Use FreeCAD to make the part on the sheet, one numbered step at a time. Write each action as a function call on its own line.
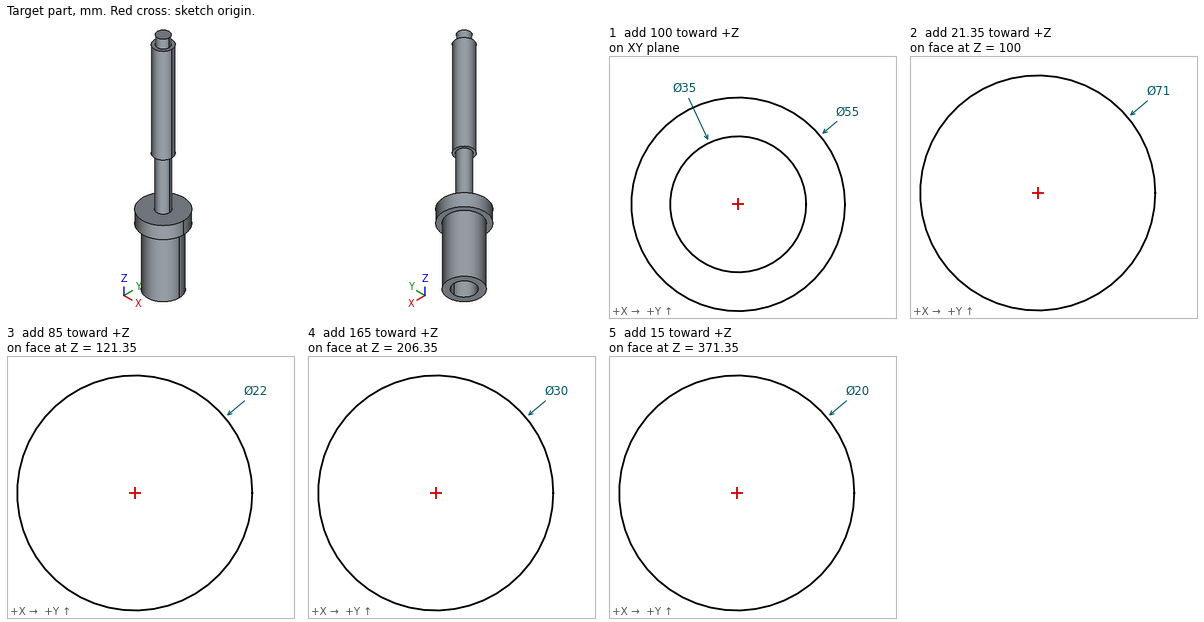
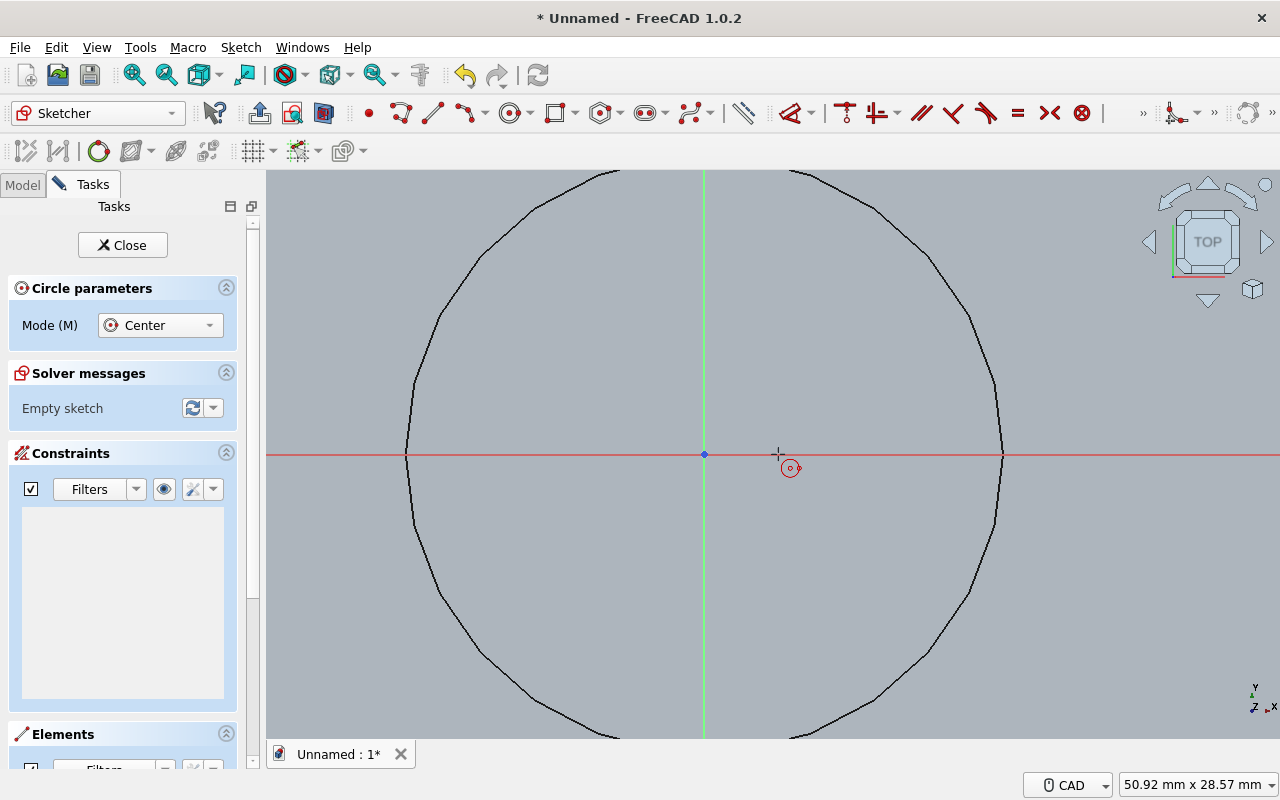
click(704, 454)
click(845, 314)
key(Escape)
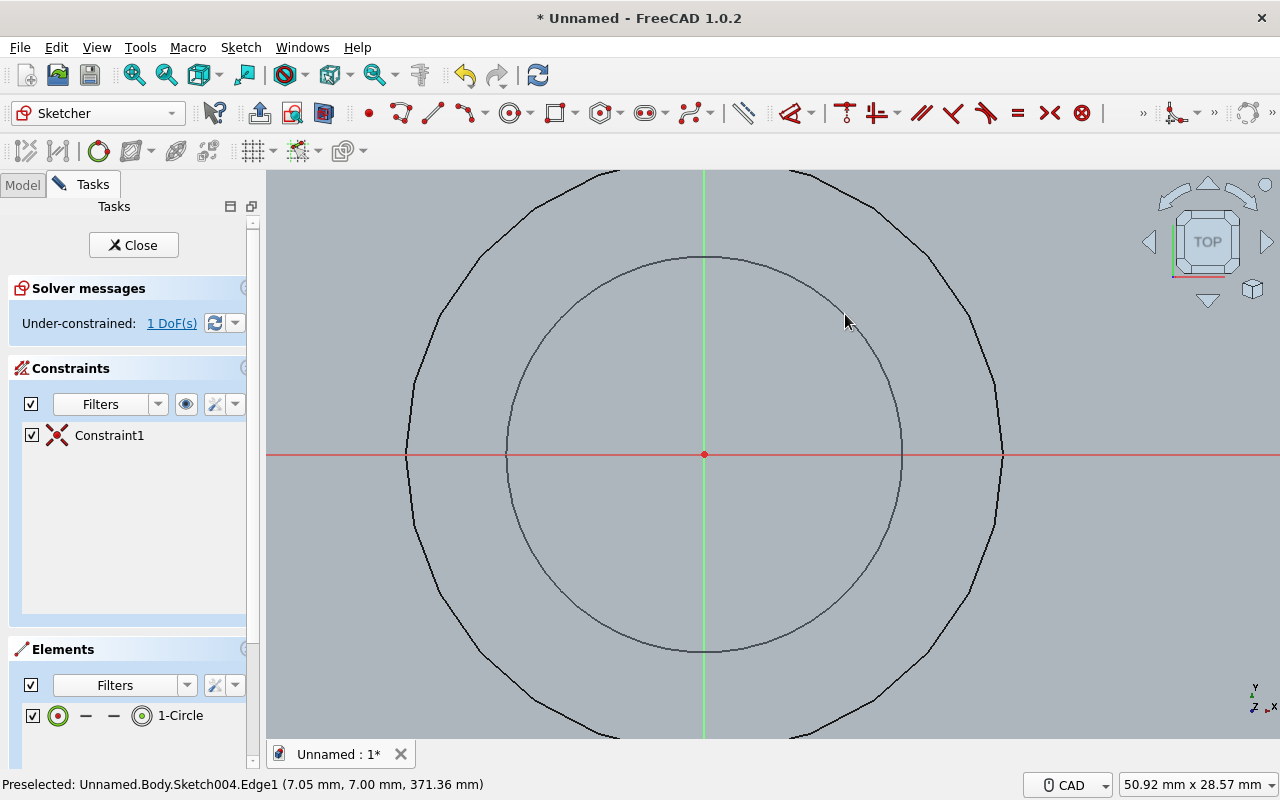
click(844, 314)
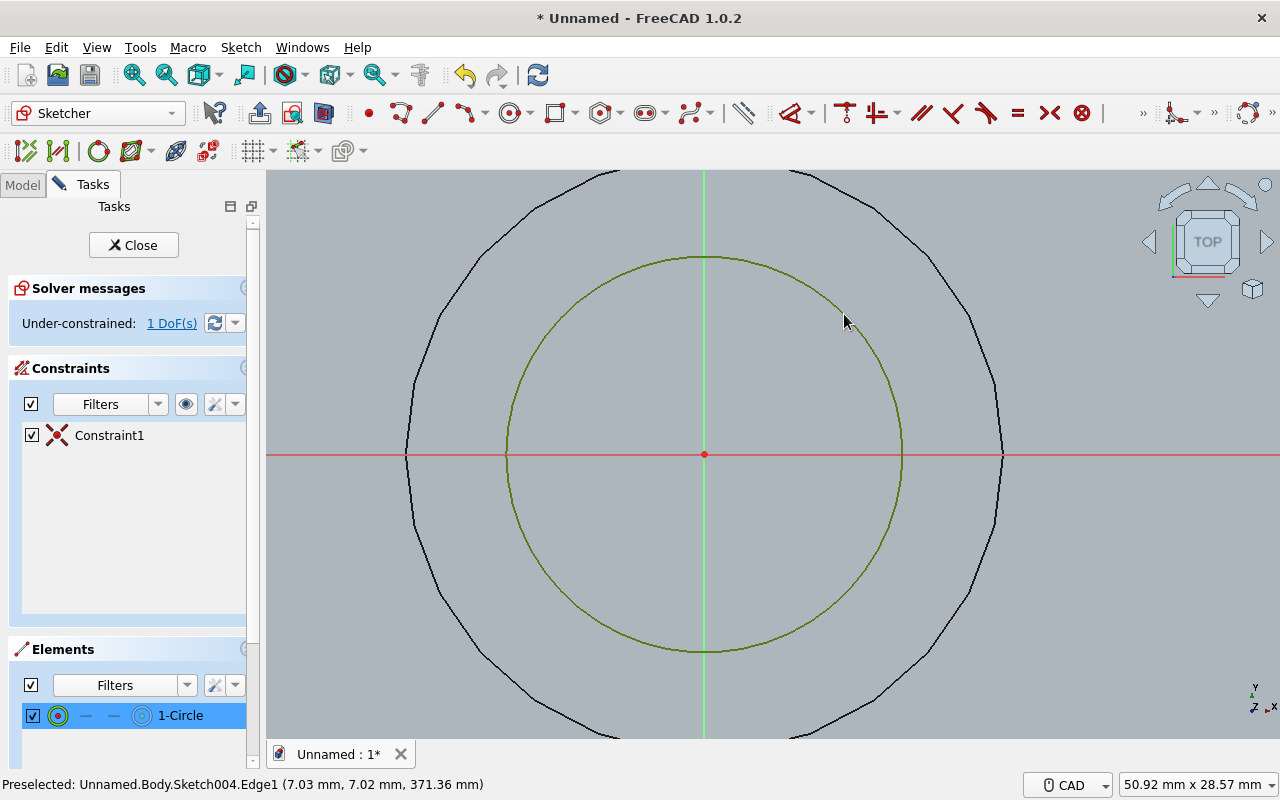
key(k)
key(o)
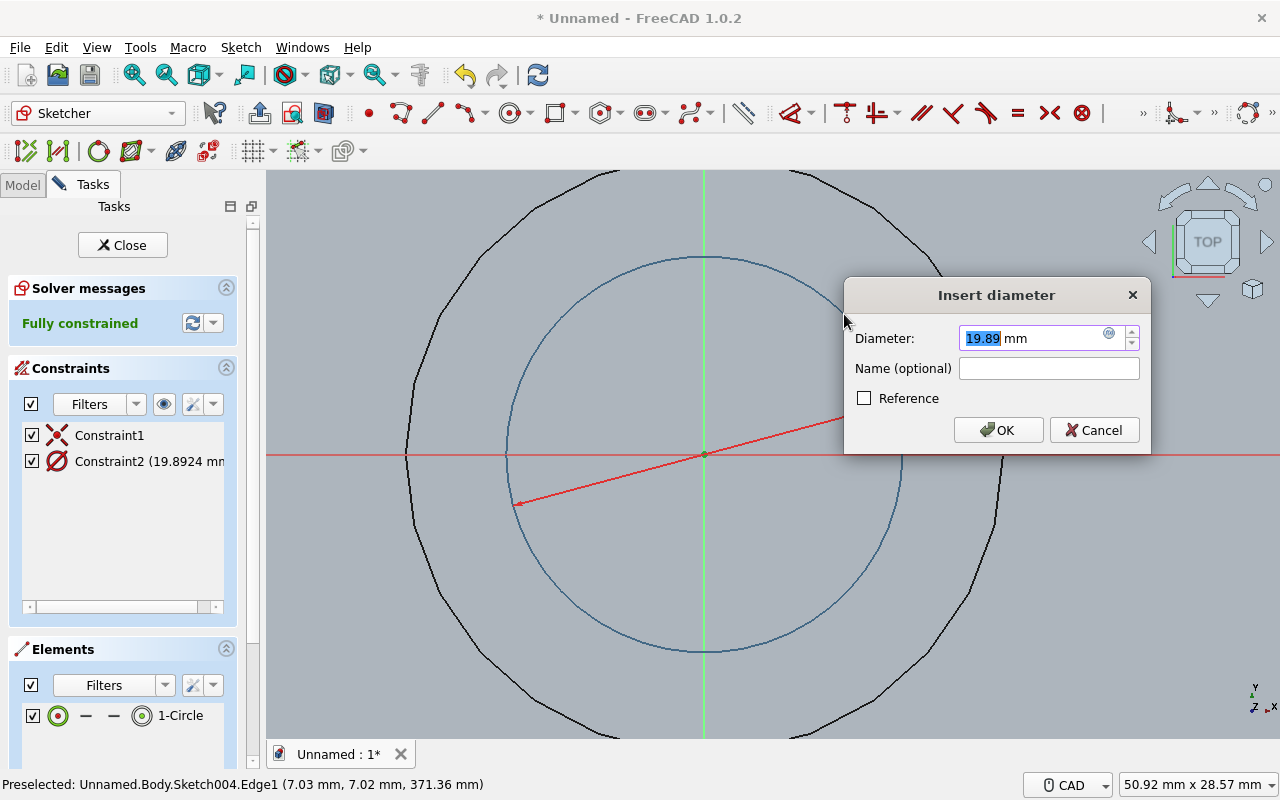
text(20)
key(Return)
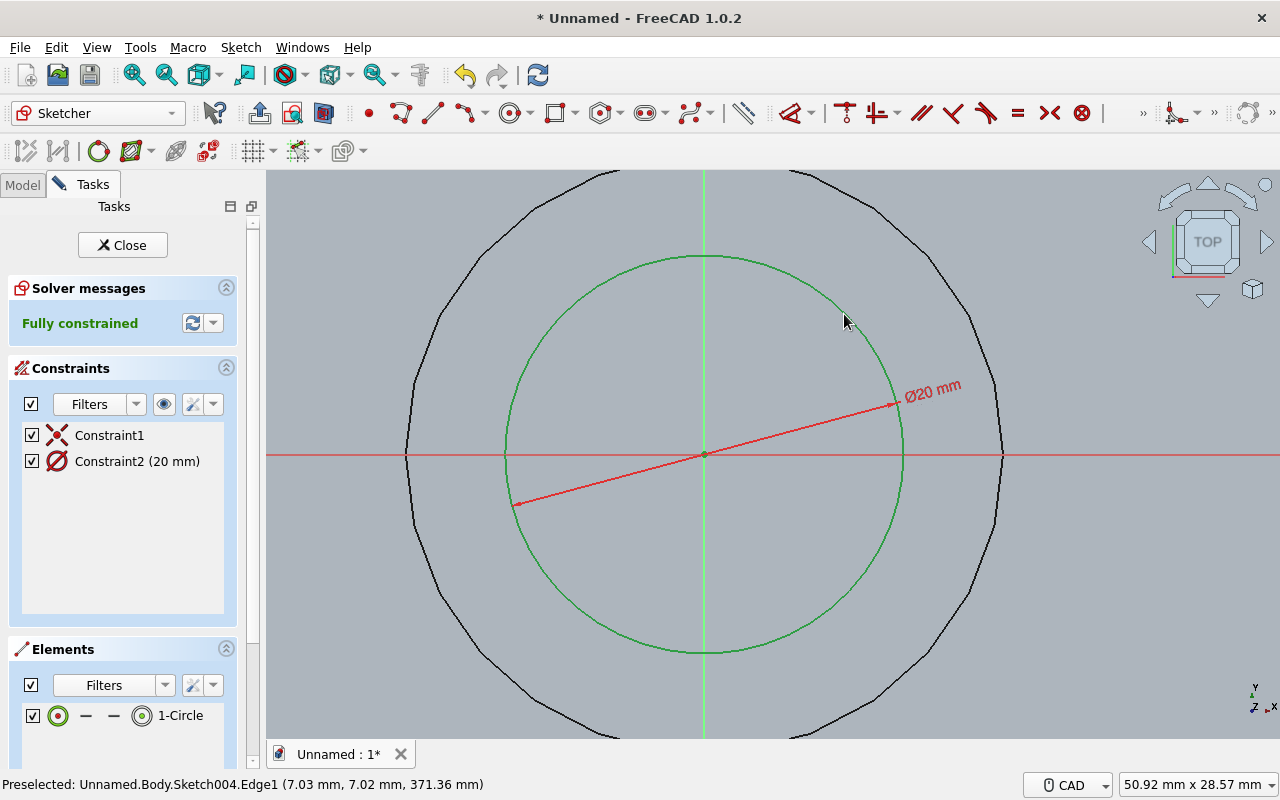
click(123, 245)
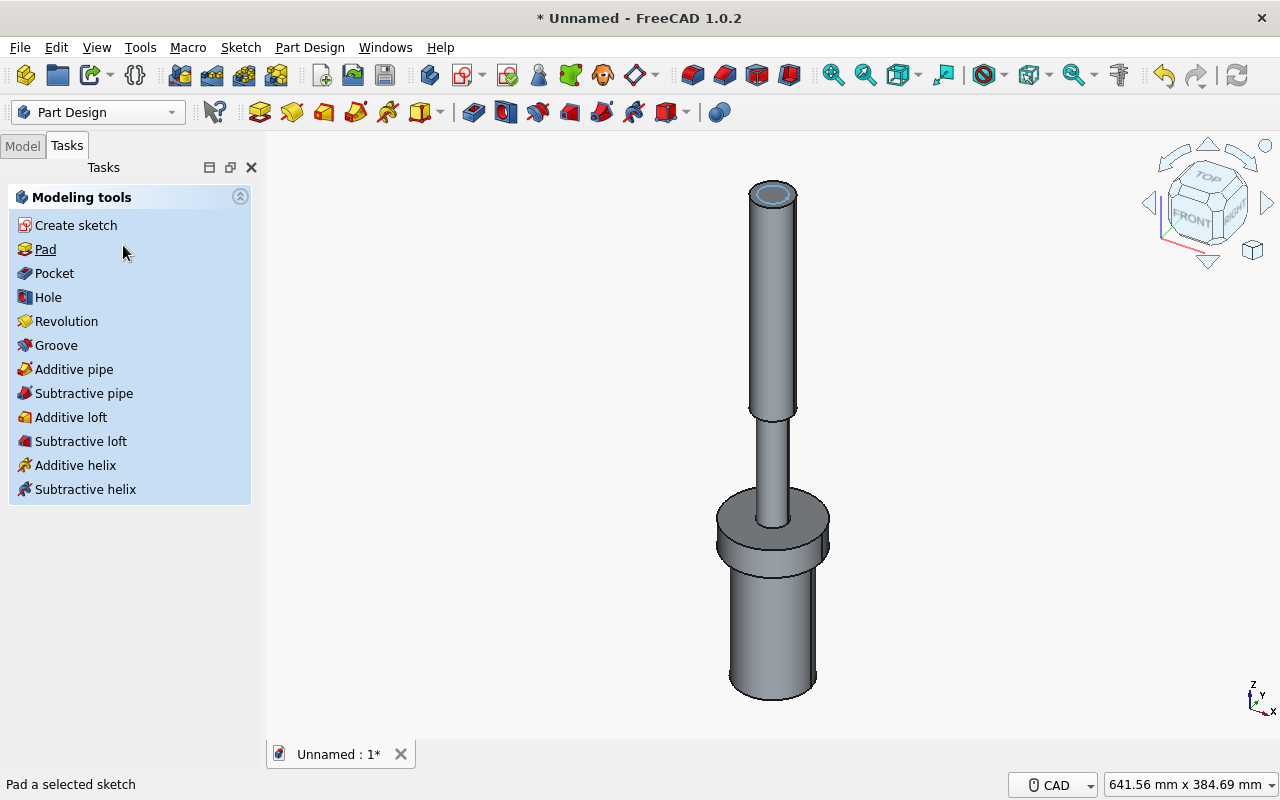
click(260, 112)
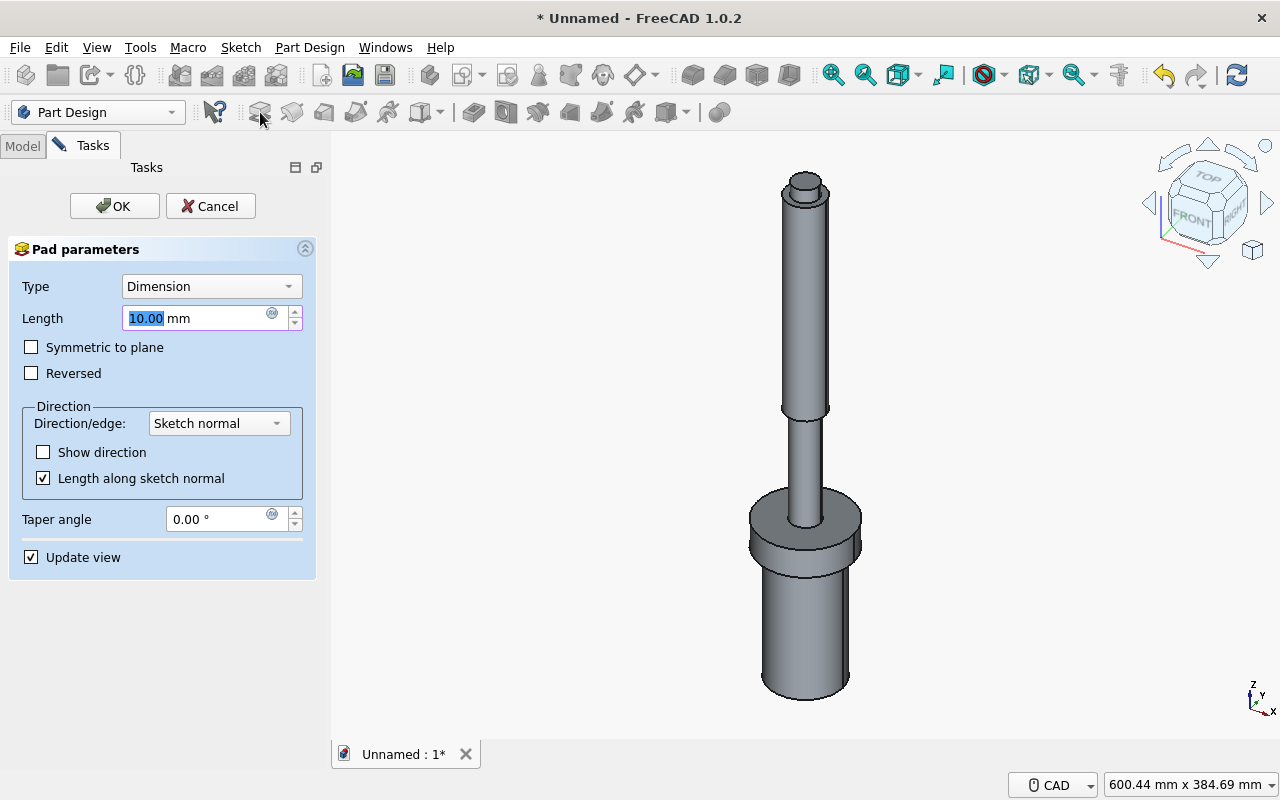
text(15)
key(Tab)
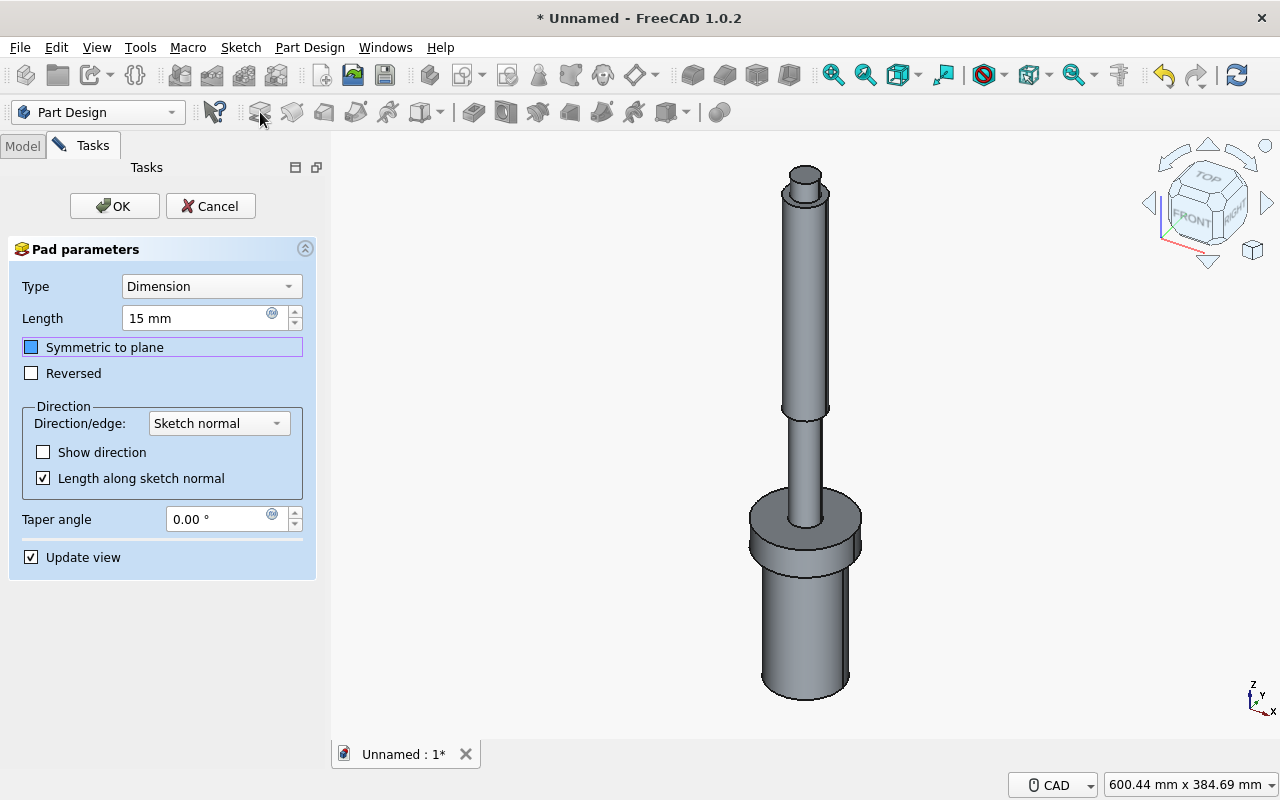
click(115, 206)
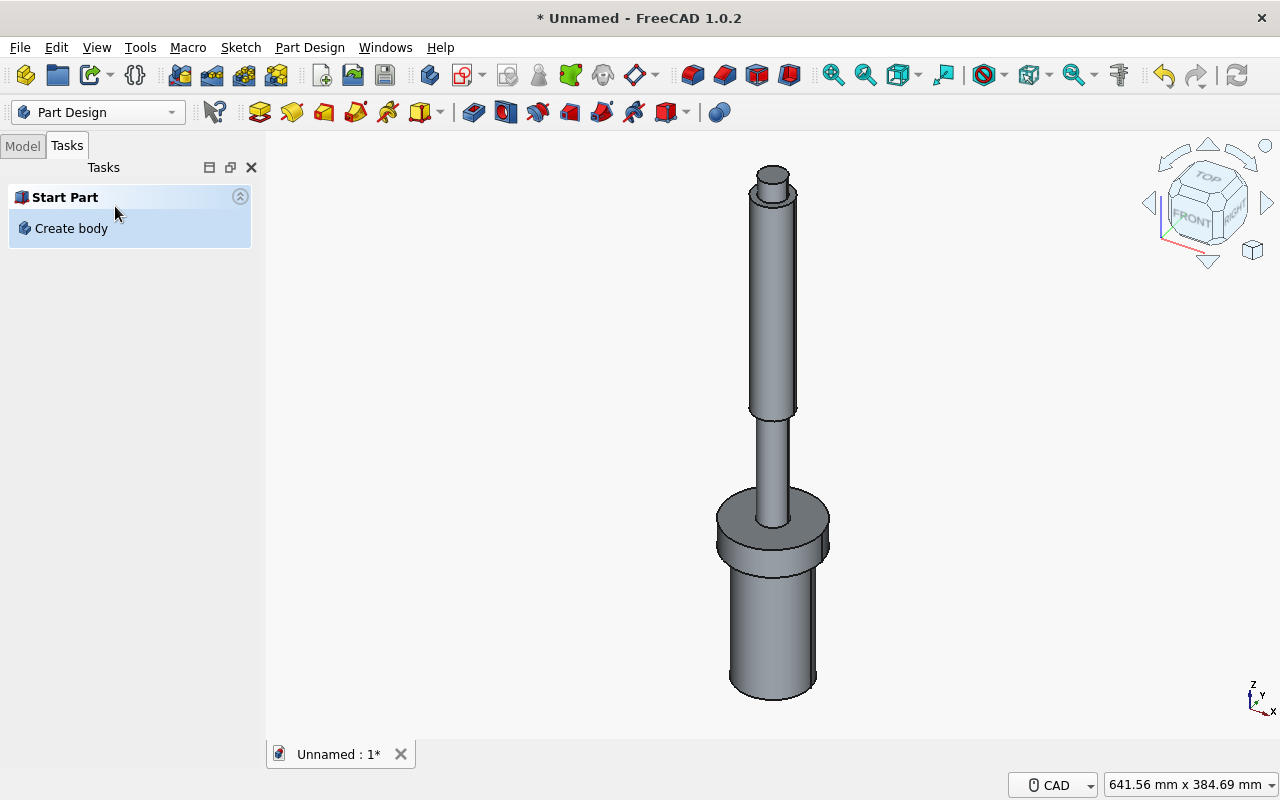
key(0)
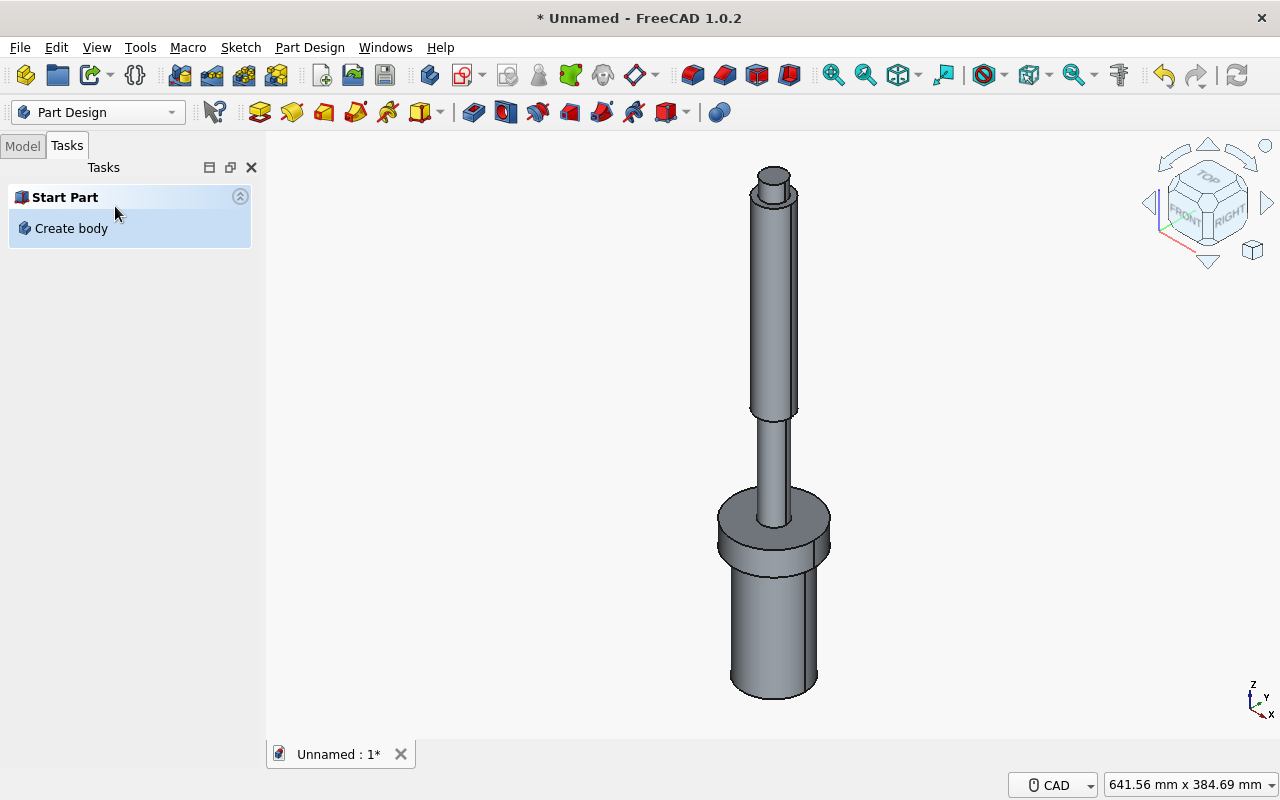
key(v)
key(f)